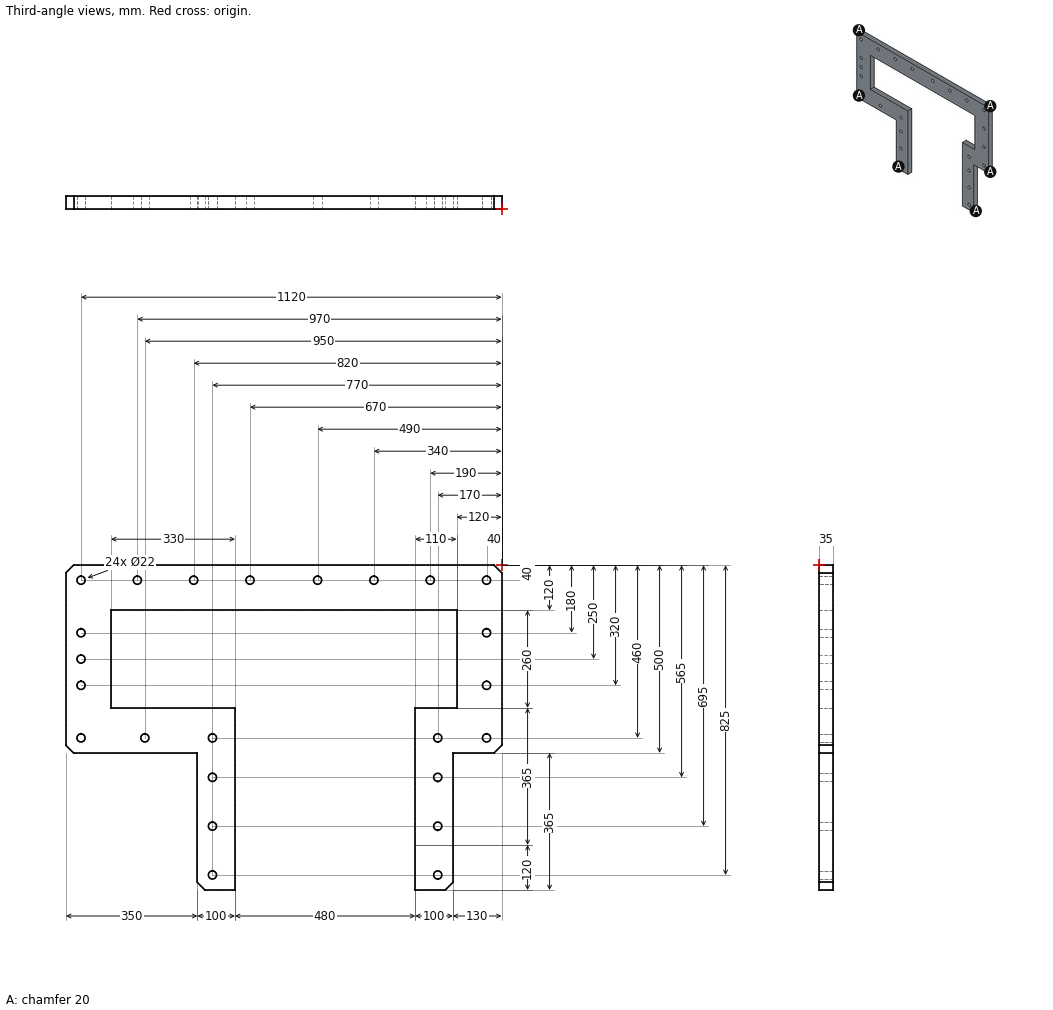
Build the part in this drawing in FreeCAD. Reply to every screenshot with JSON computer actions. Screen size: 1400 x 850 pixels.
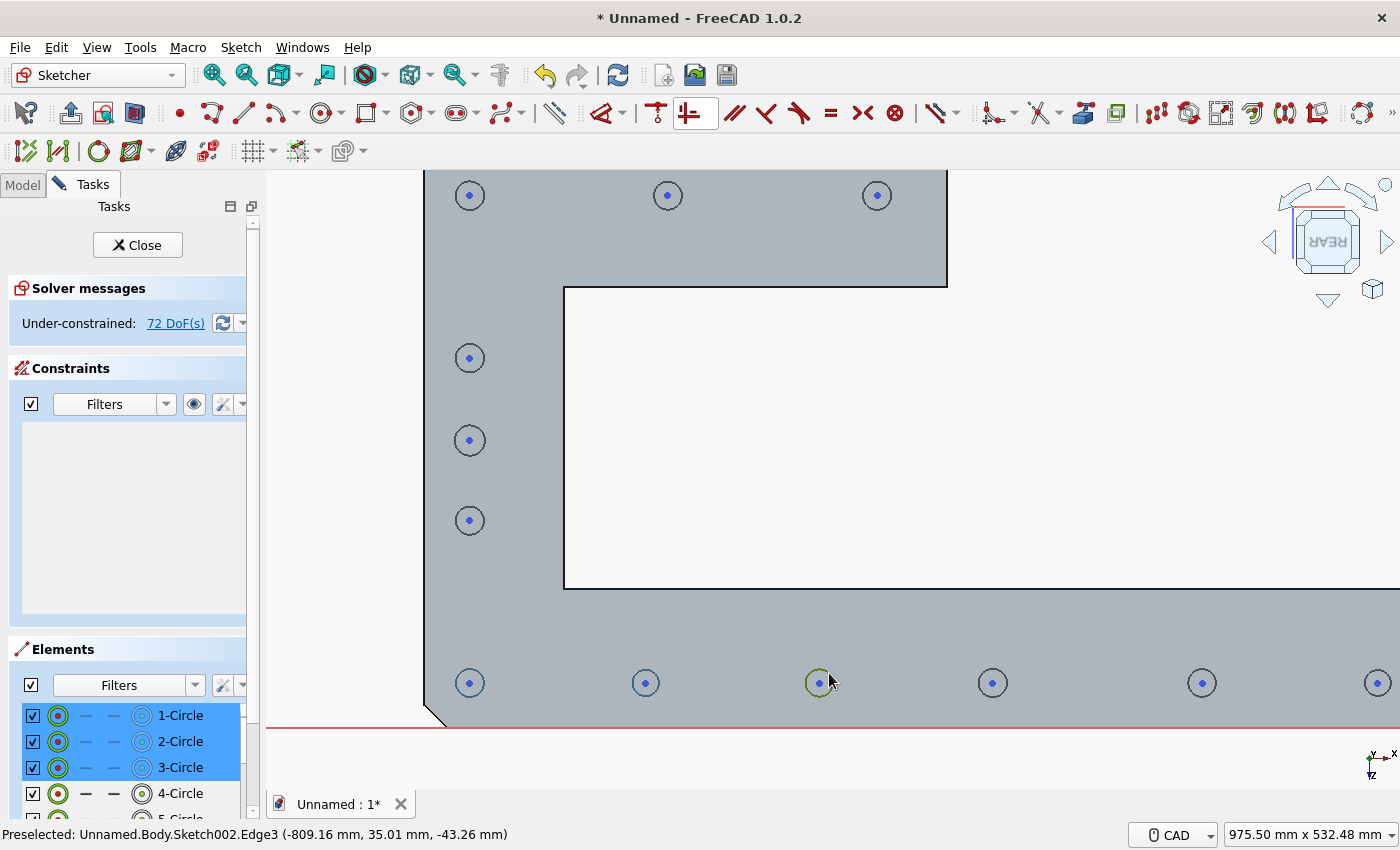
{"action": "left_click", "coordinate": [1003, 673]}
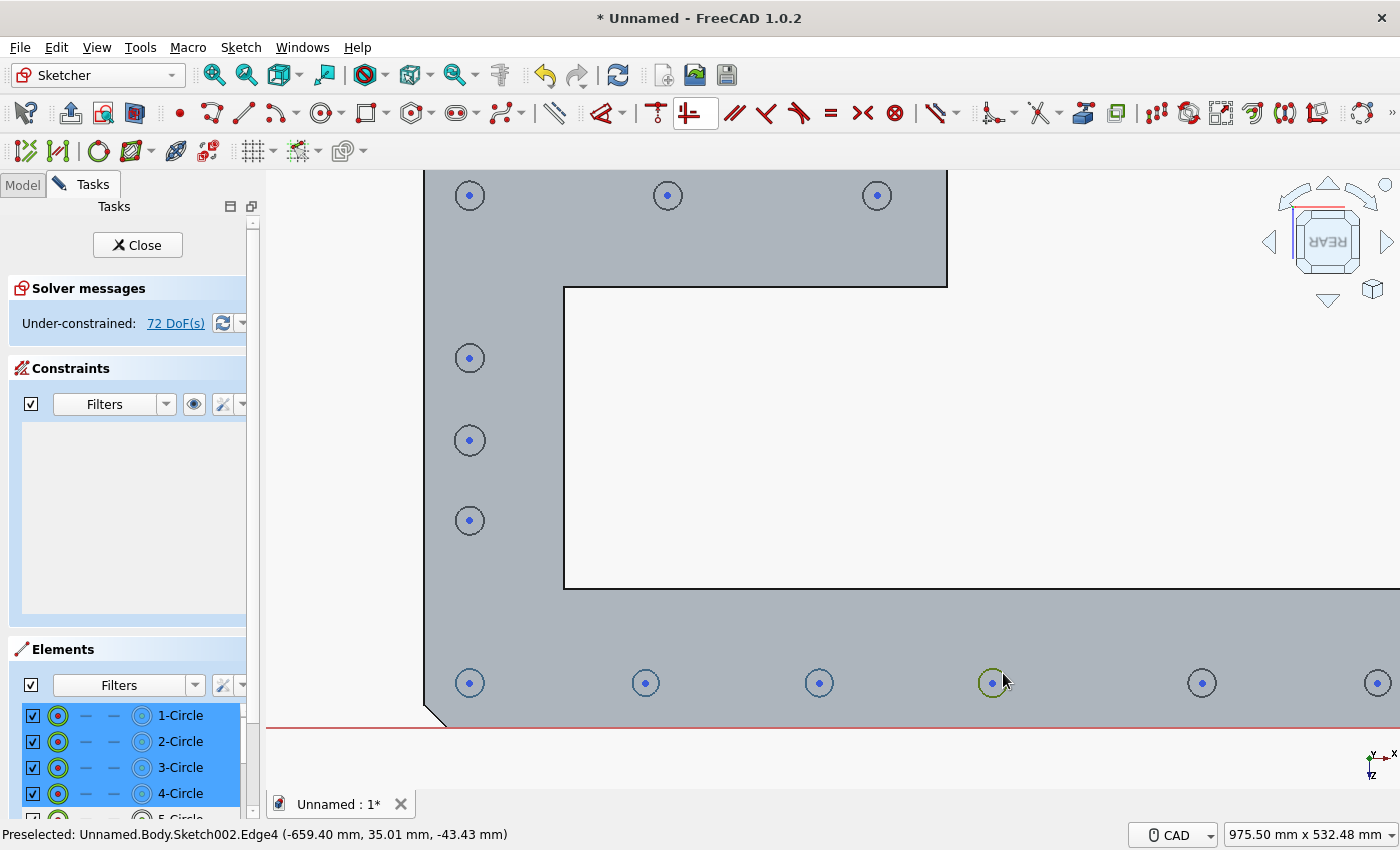
{"action": "left_click", "coordinate": [1212, 673]}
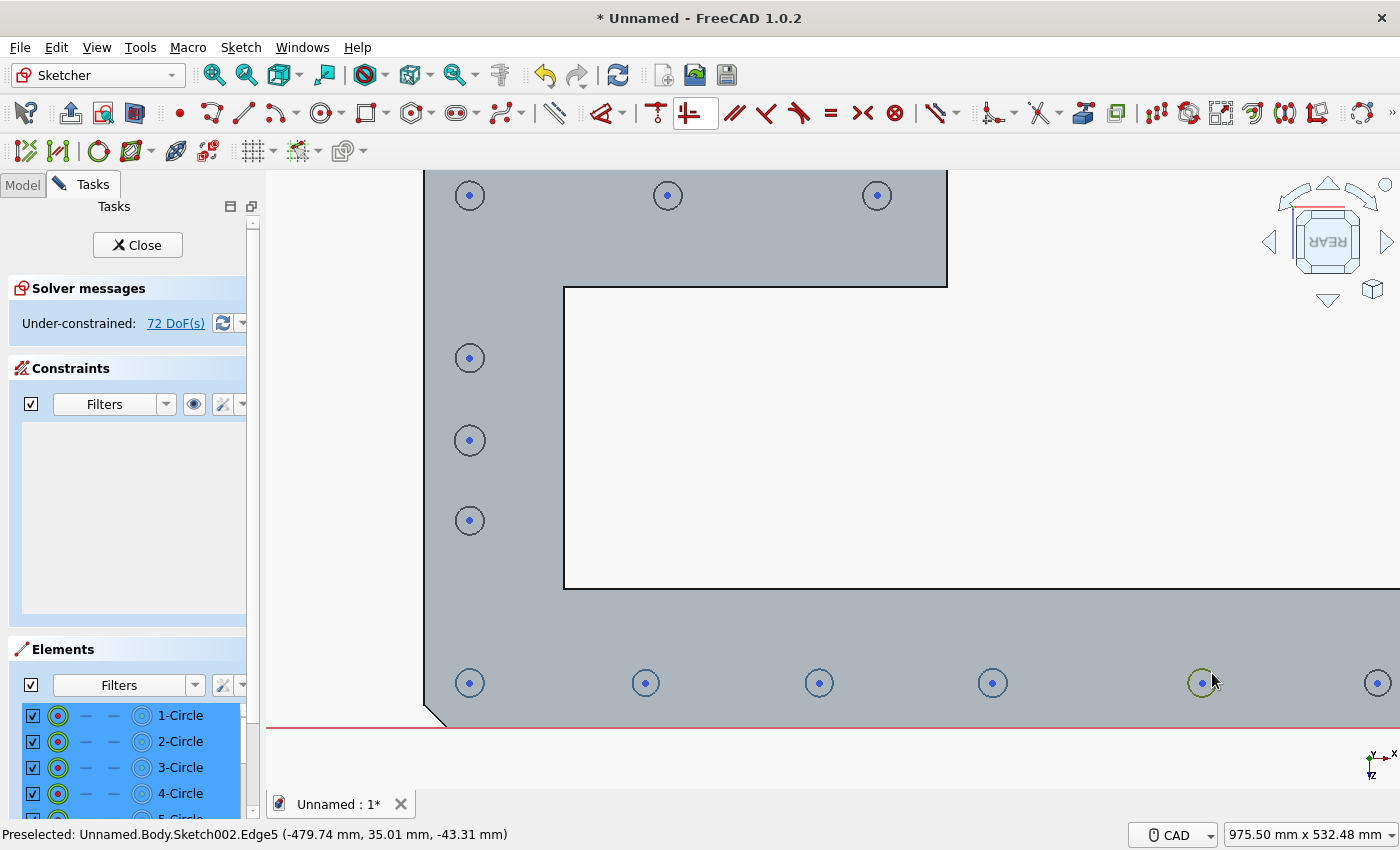
{"action": "scroll", "coordinate": [478, 673], "scroll_direction": "down", "scroll_amount": 4}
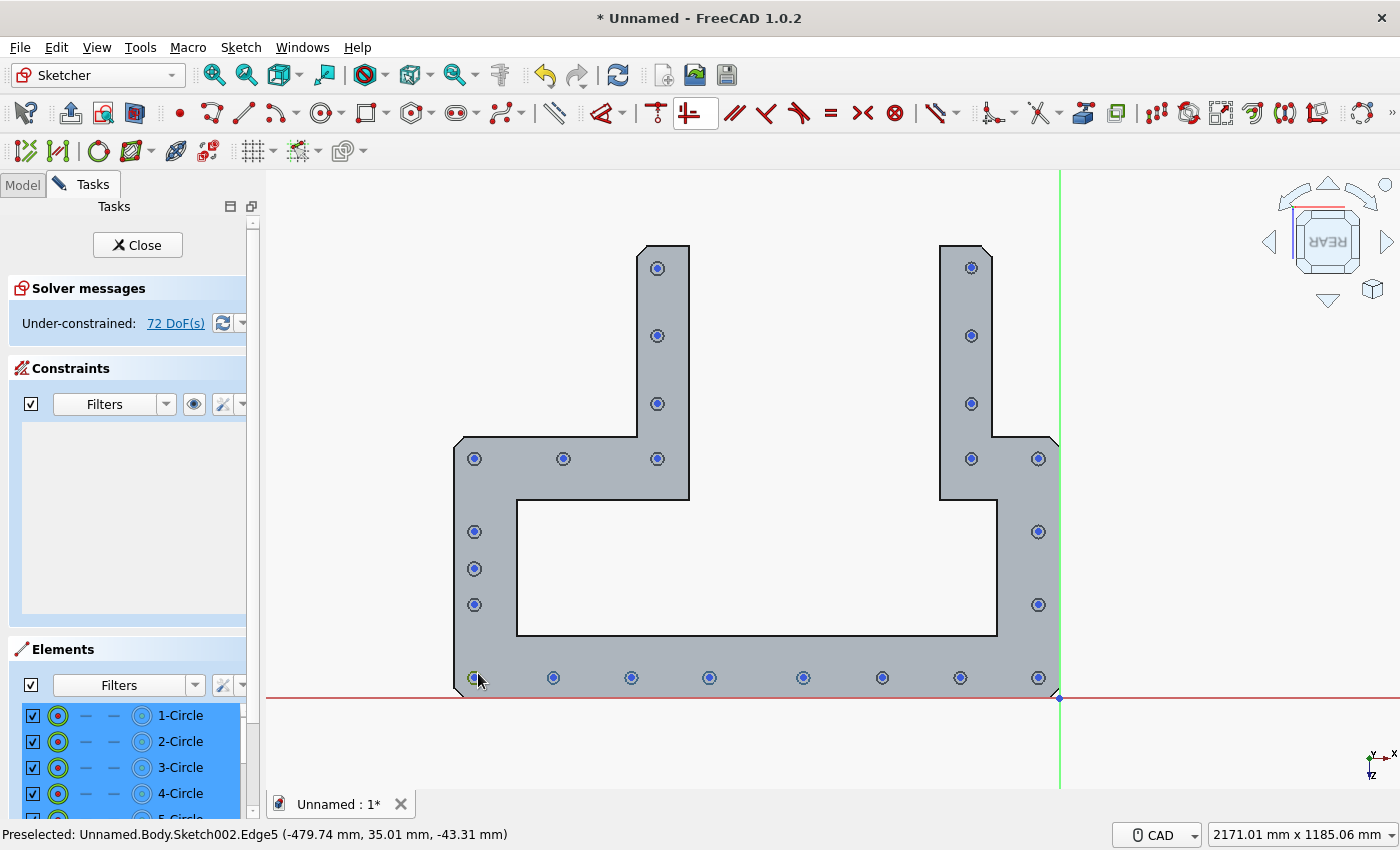
{"action": "scroll", "coordinate": [887, 674], "scroll_direction": "up", "scroll_amount": 5}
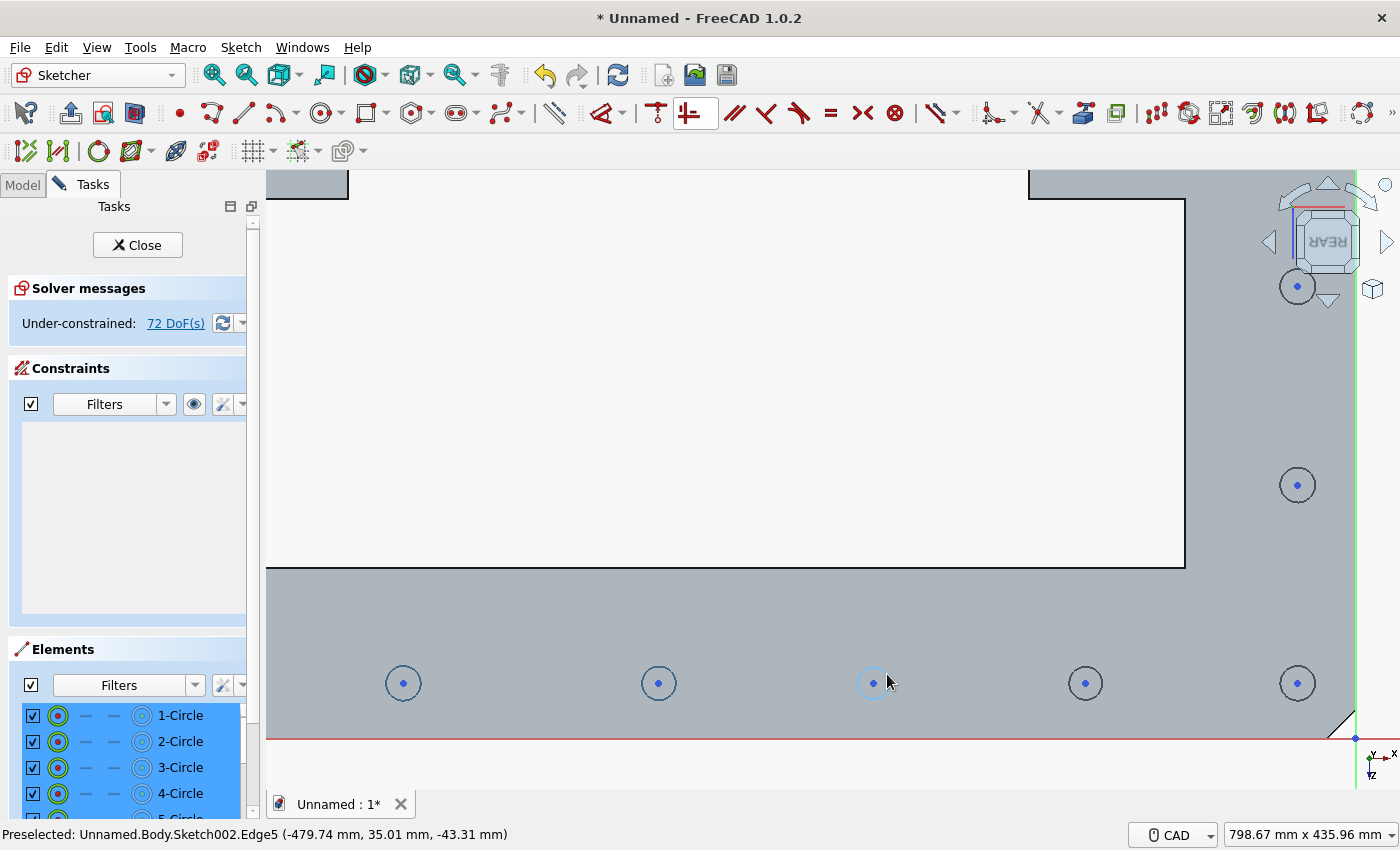
{"action": "left_click", "coordinate": [885, 672]}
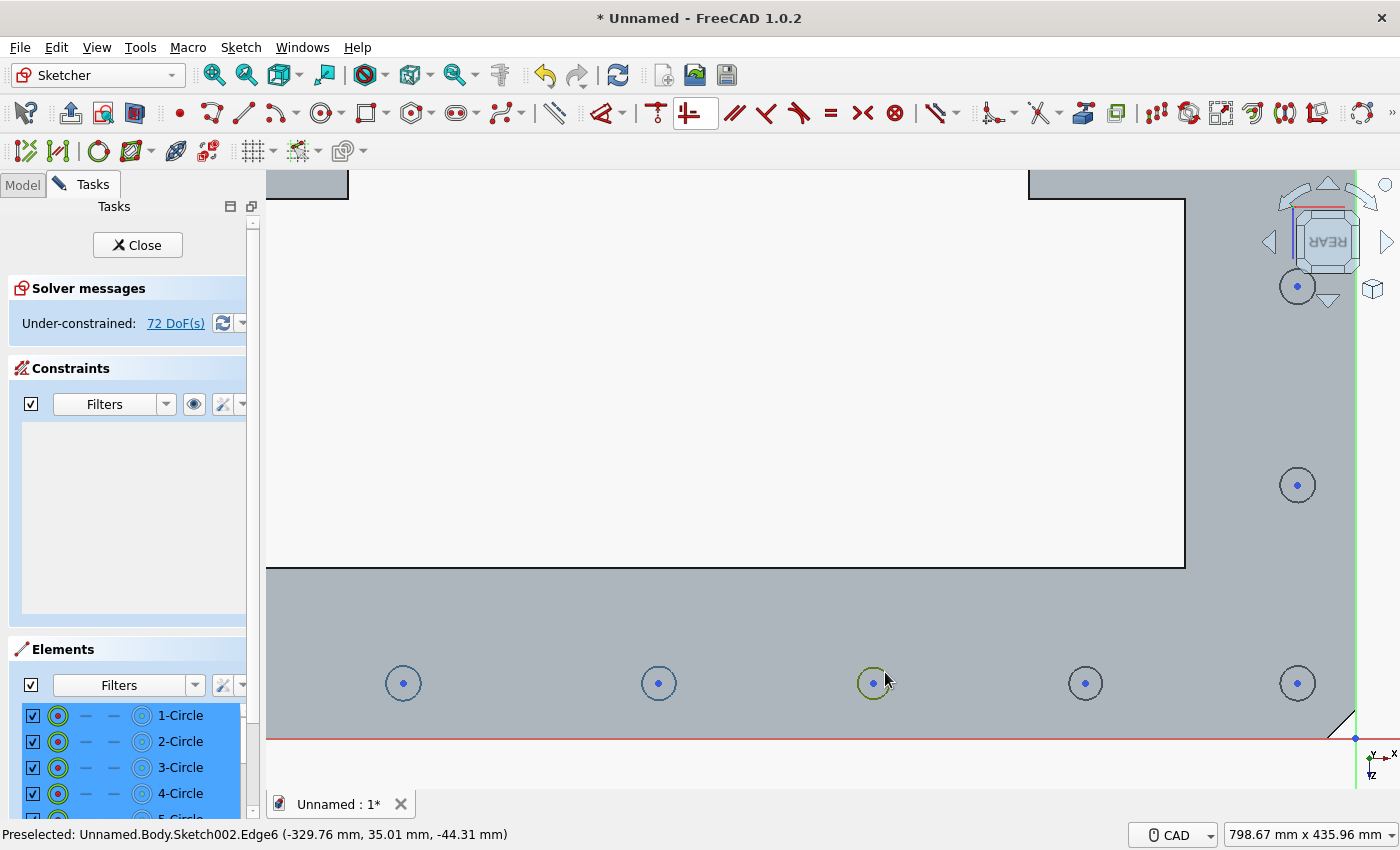
{"action": "left_click", "coordinate": [1097, 672]}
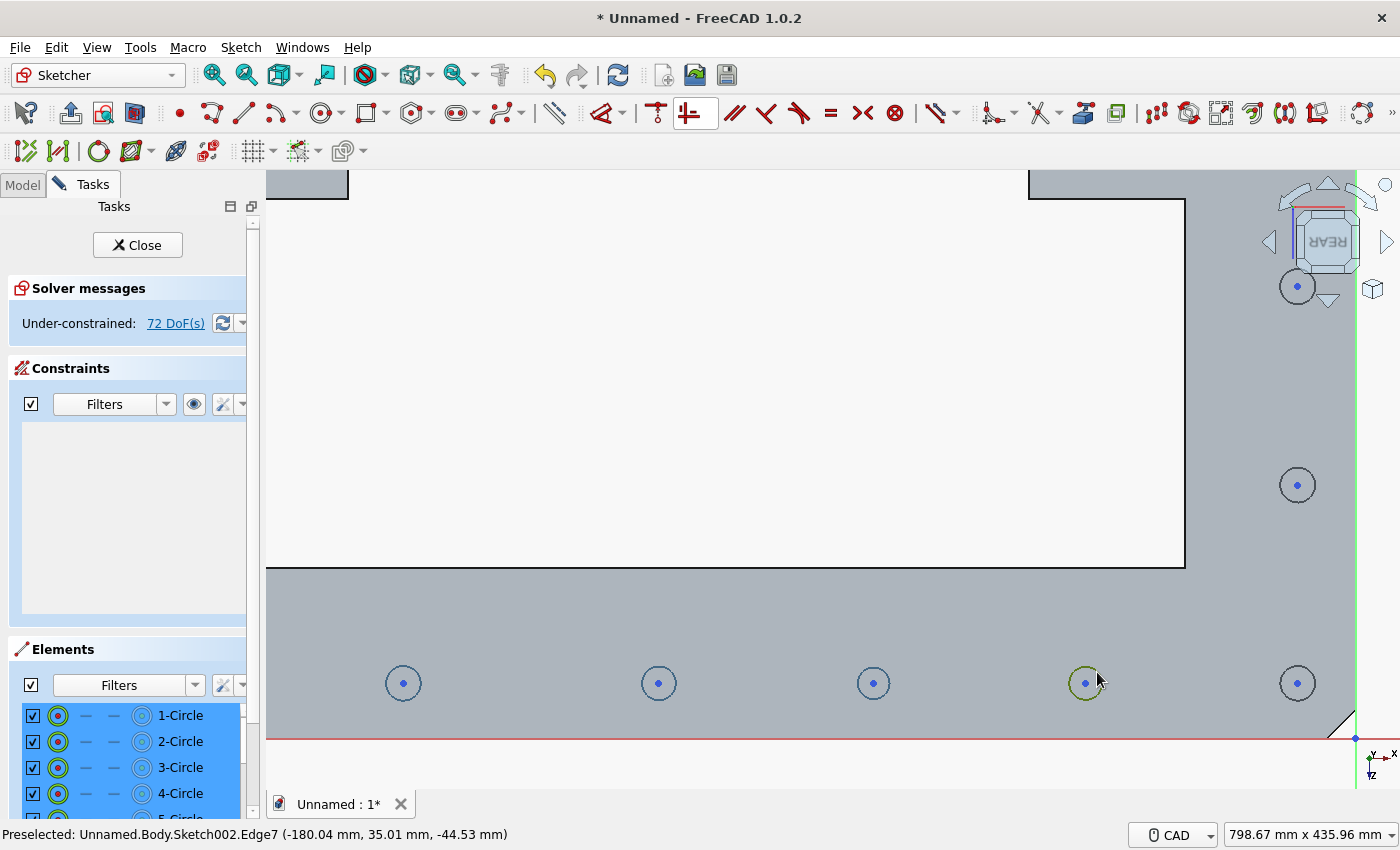
{"action": "scroll", "coordinate": [888, 674], "scroll_direction": "down", "scroll_amount": 5}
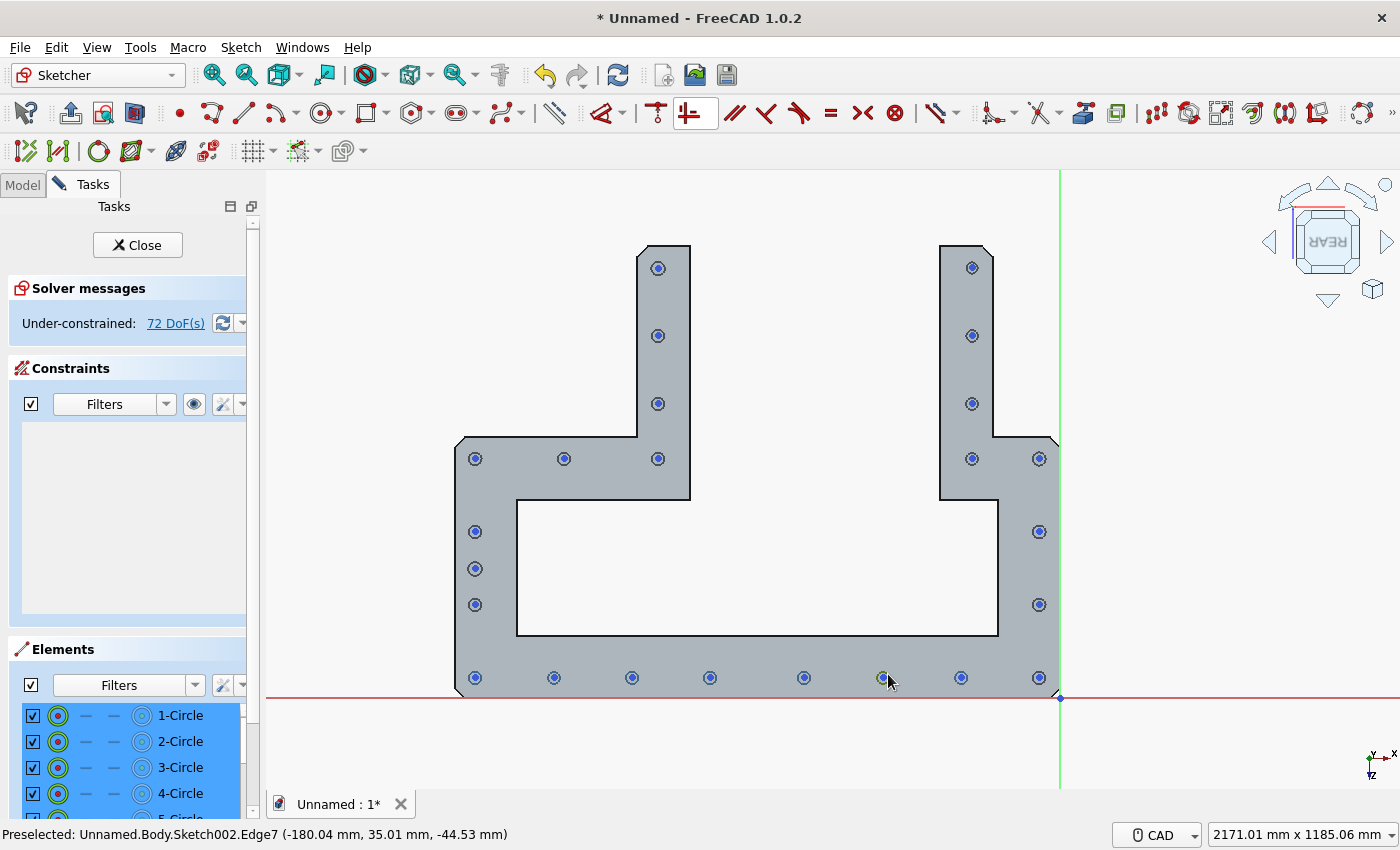
{"action": "scroll", "coordinate": [1044, 673], "scroll_direction": "up", "scroll_amount": 4}